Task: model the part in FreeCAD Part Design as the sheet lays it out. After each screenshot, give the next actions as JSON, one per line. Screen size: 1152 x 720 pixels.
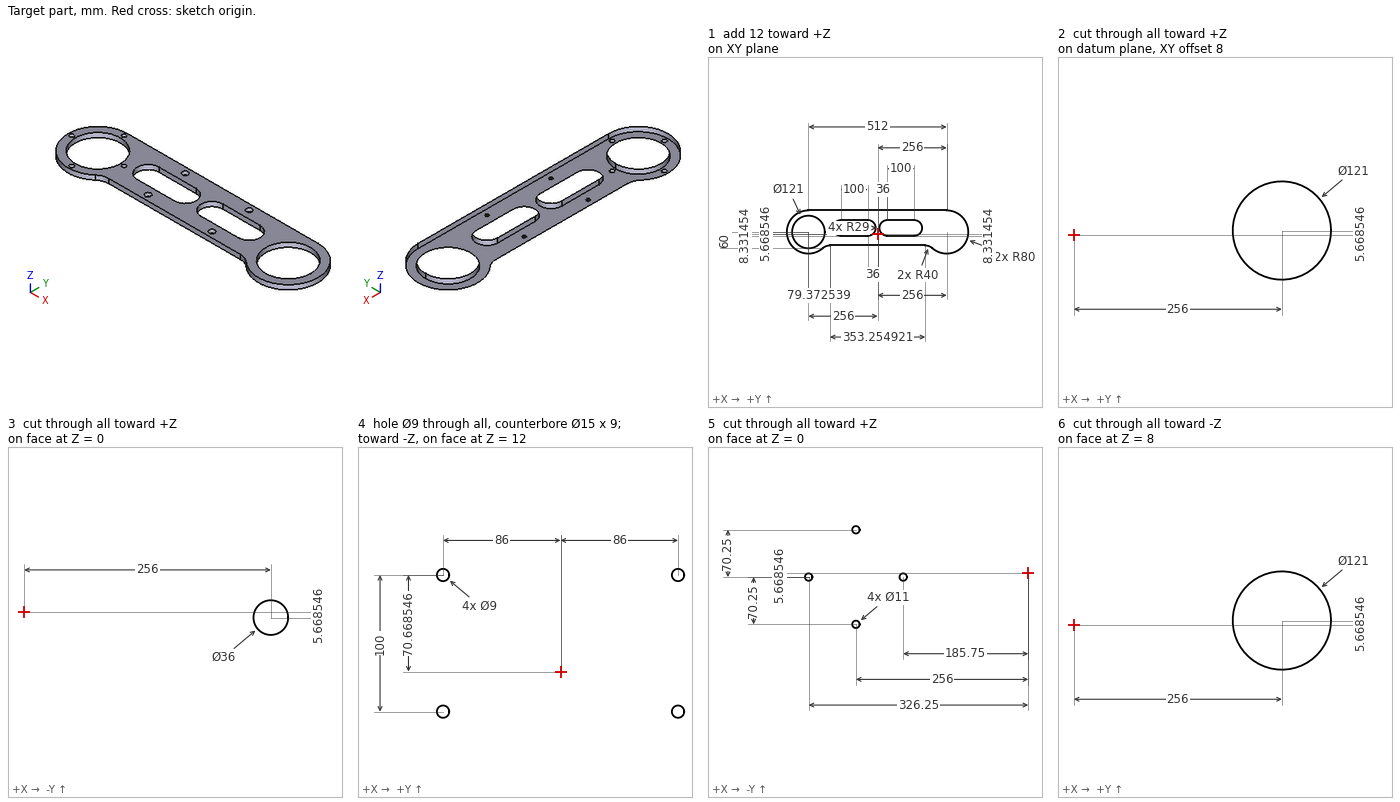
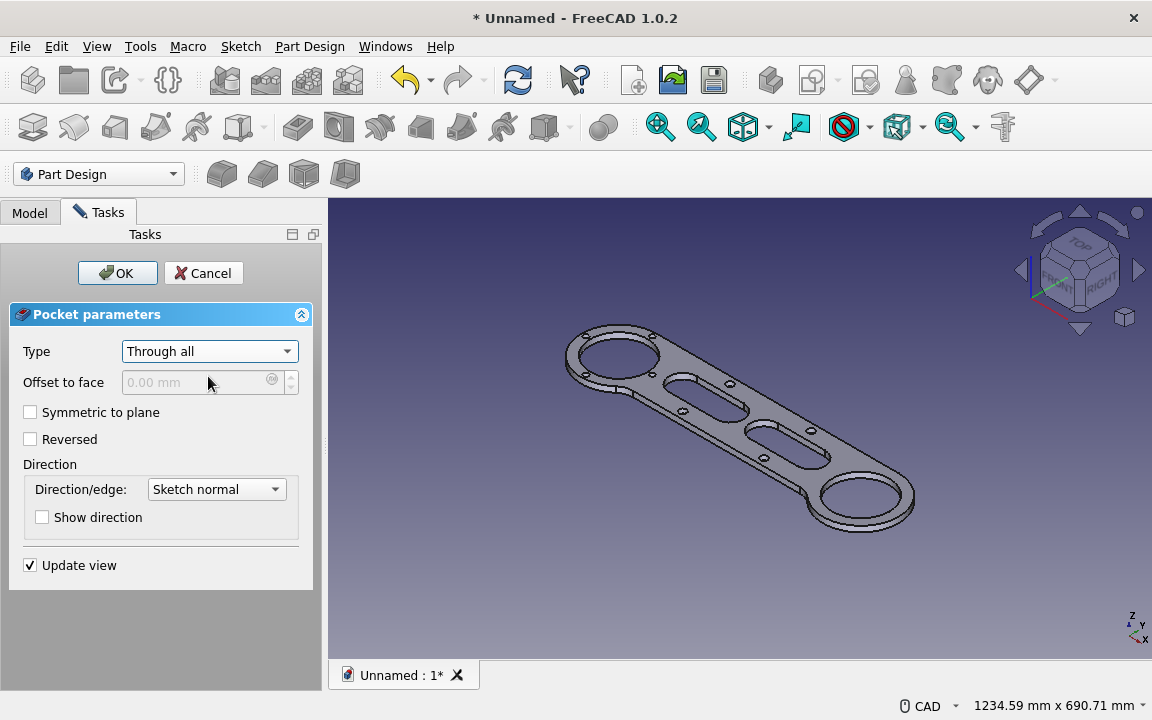
{"action": "left_click", "coordinate": [118, 273]}